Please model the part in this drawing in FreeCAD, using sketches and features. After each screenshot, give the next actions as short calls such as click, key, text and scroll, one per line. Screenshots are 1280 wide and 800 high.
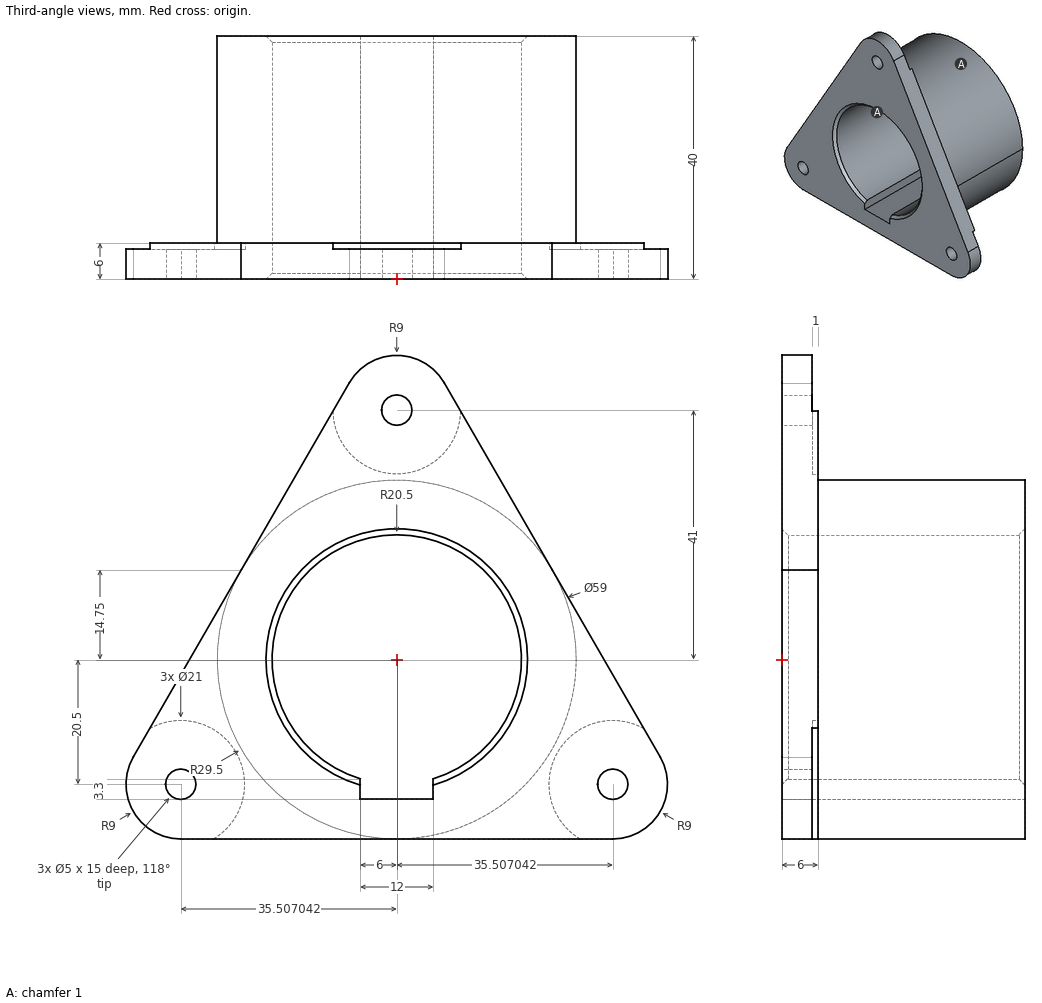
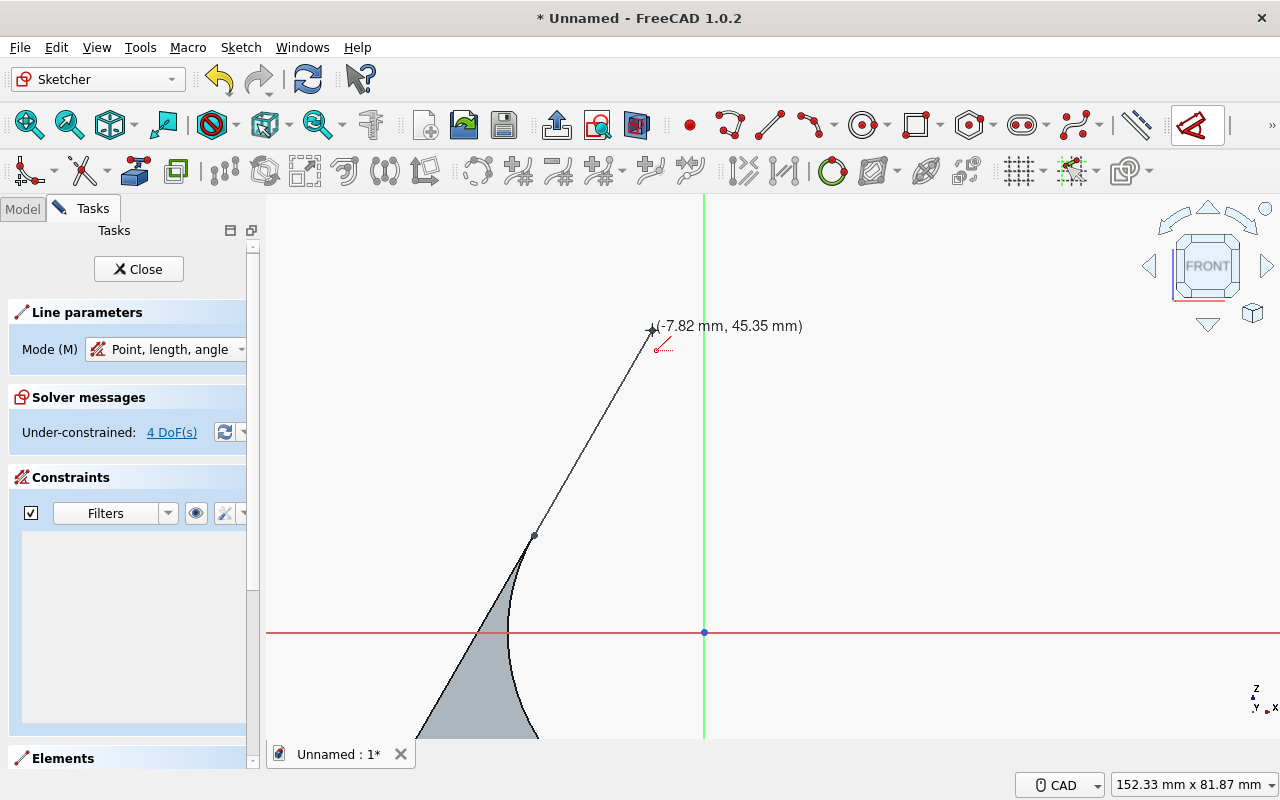
click(756, 330)
click(874, 535)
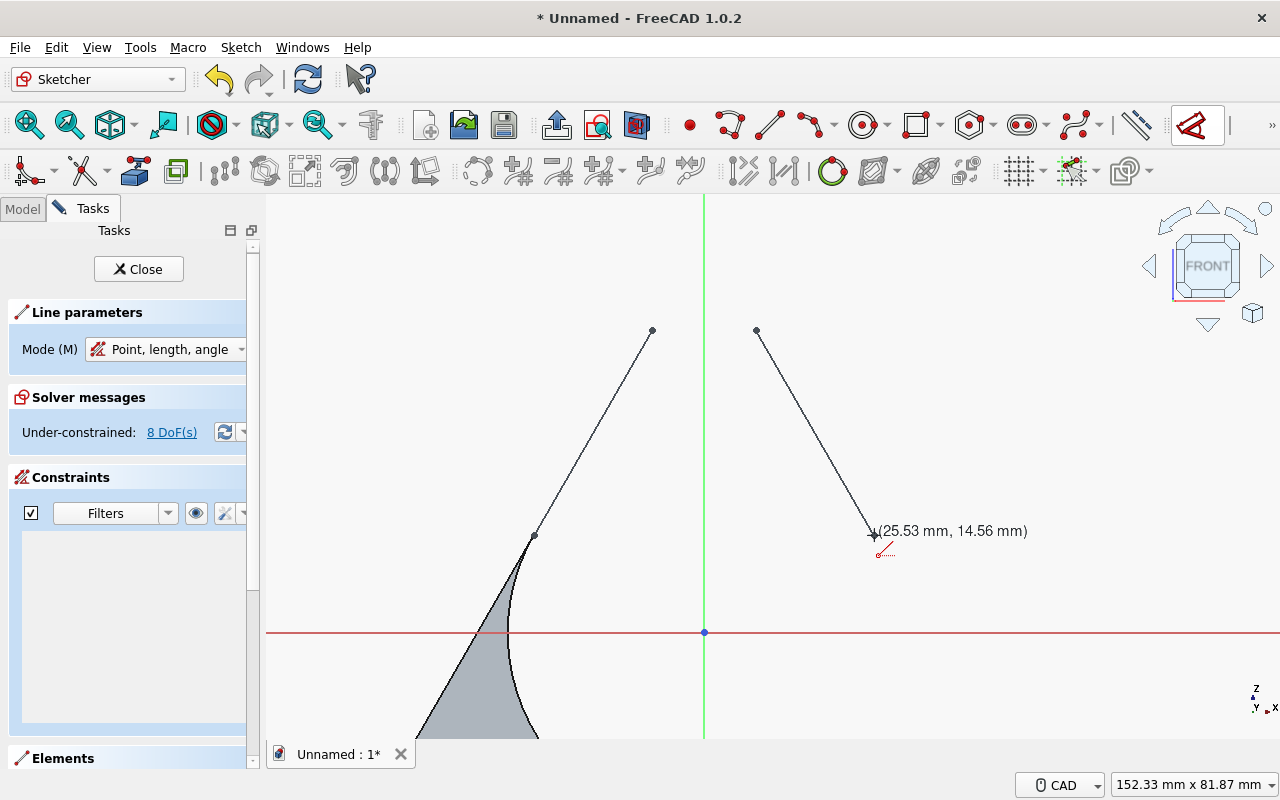
click(810, 126)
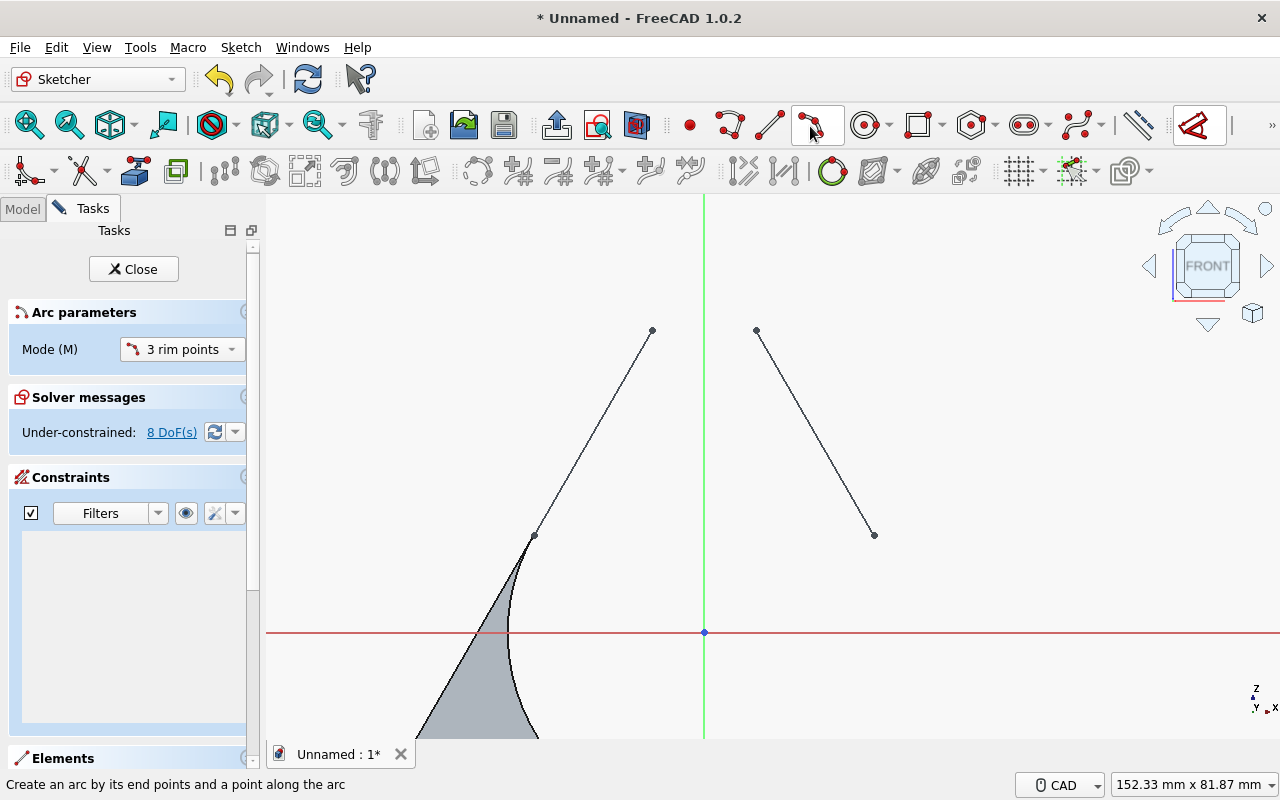
click(652, 331)
click(756, 331)
click(728, 305)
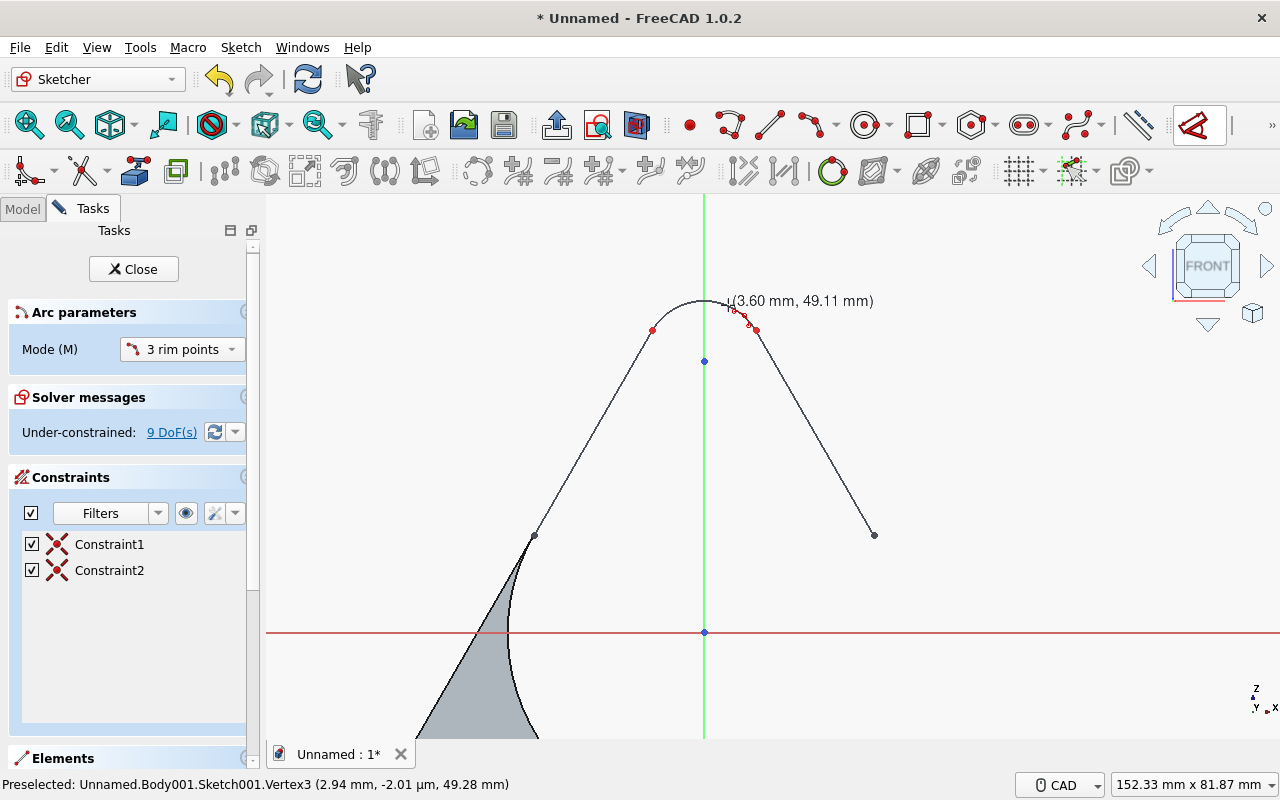
click(874, 536)
click(534, 536)
click(745, 441)
key(Escape)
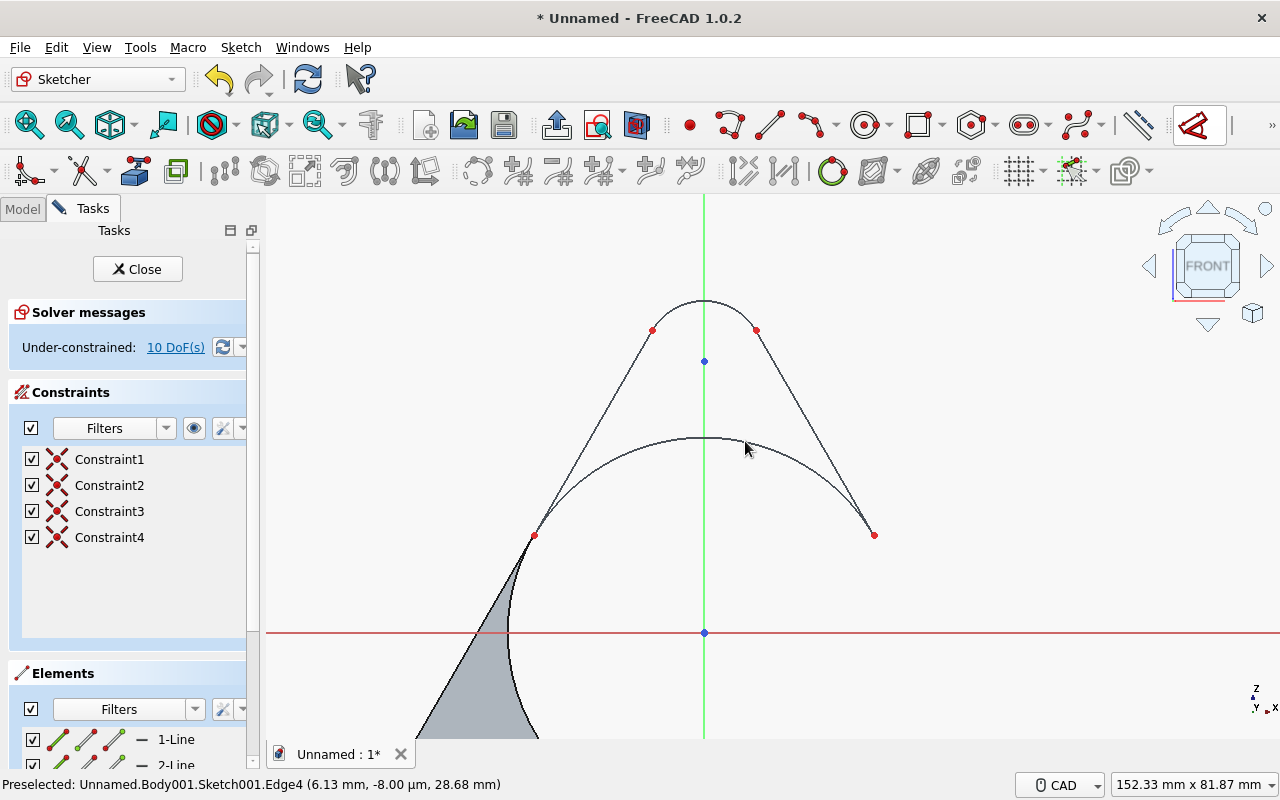
click(569, 474)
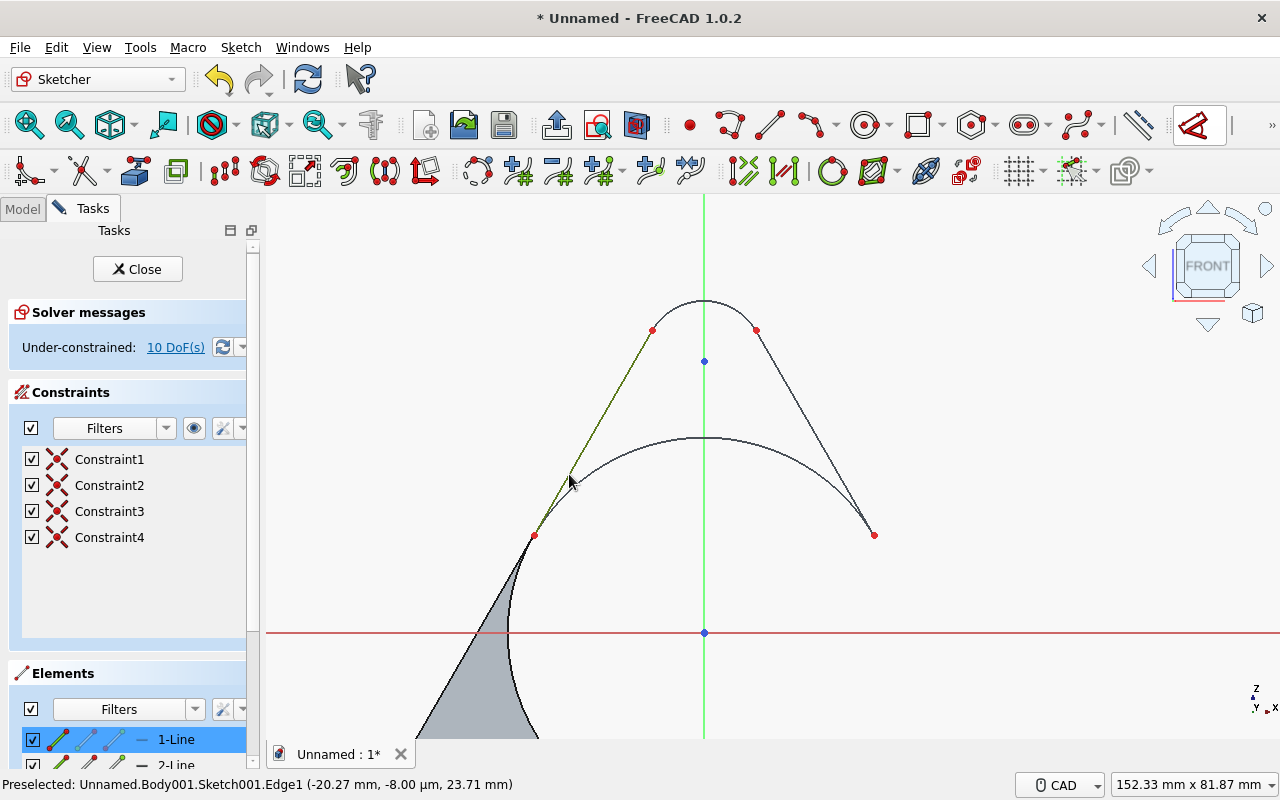
click(728, 306)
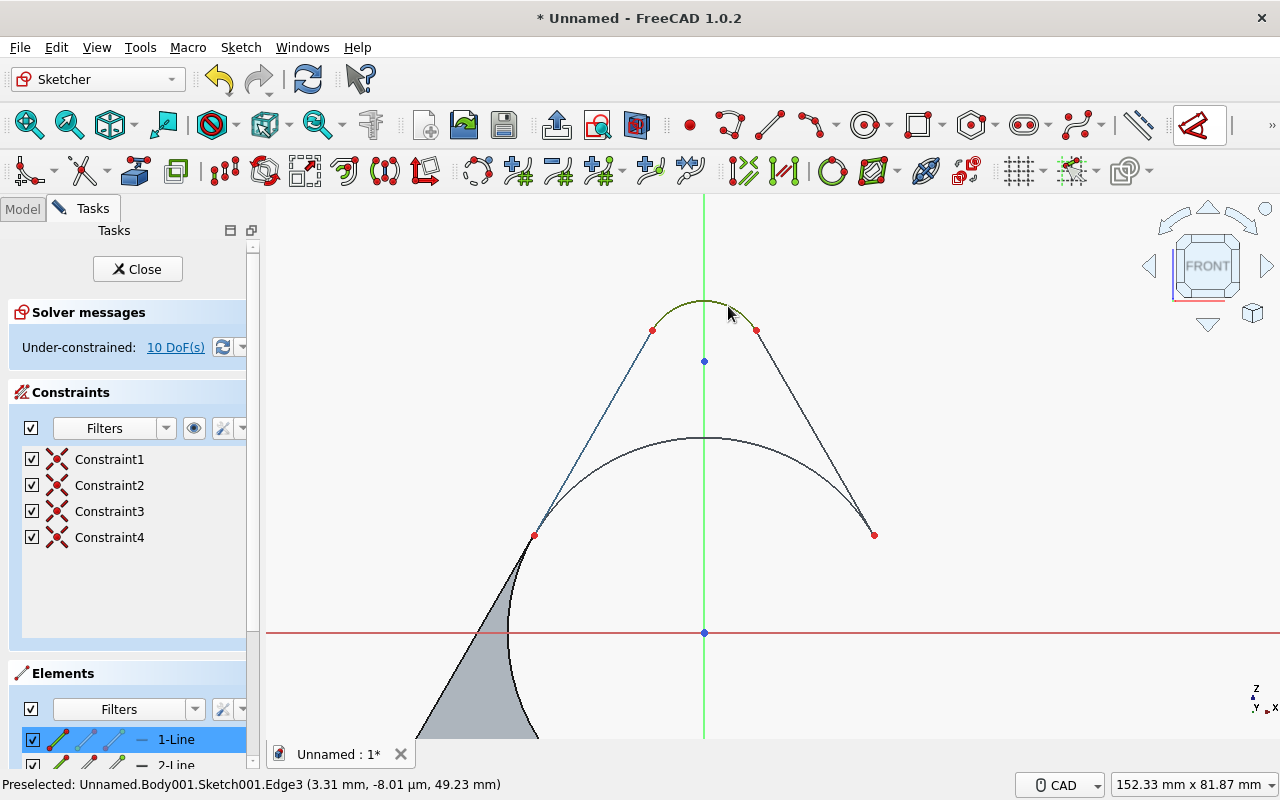
key(t)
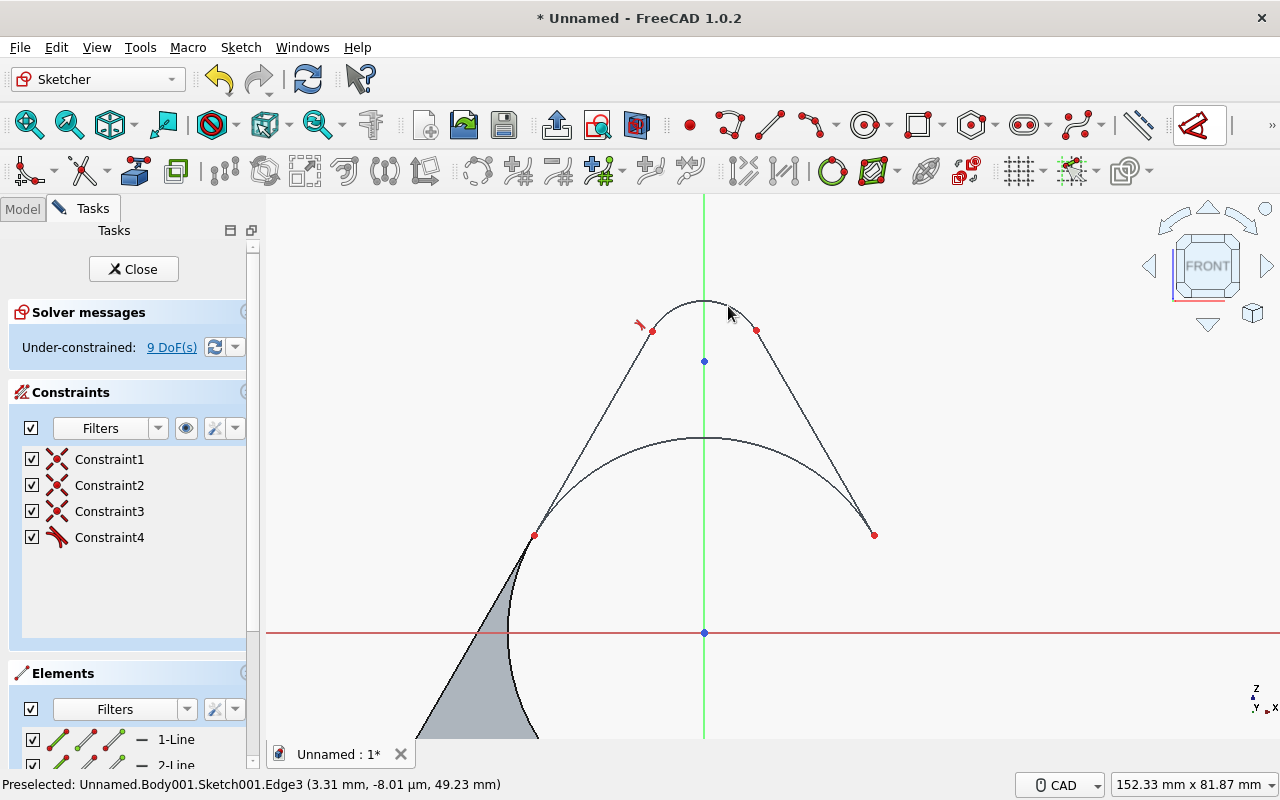
click(569, 475)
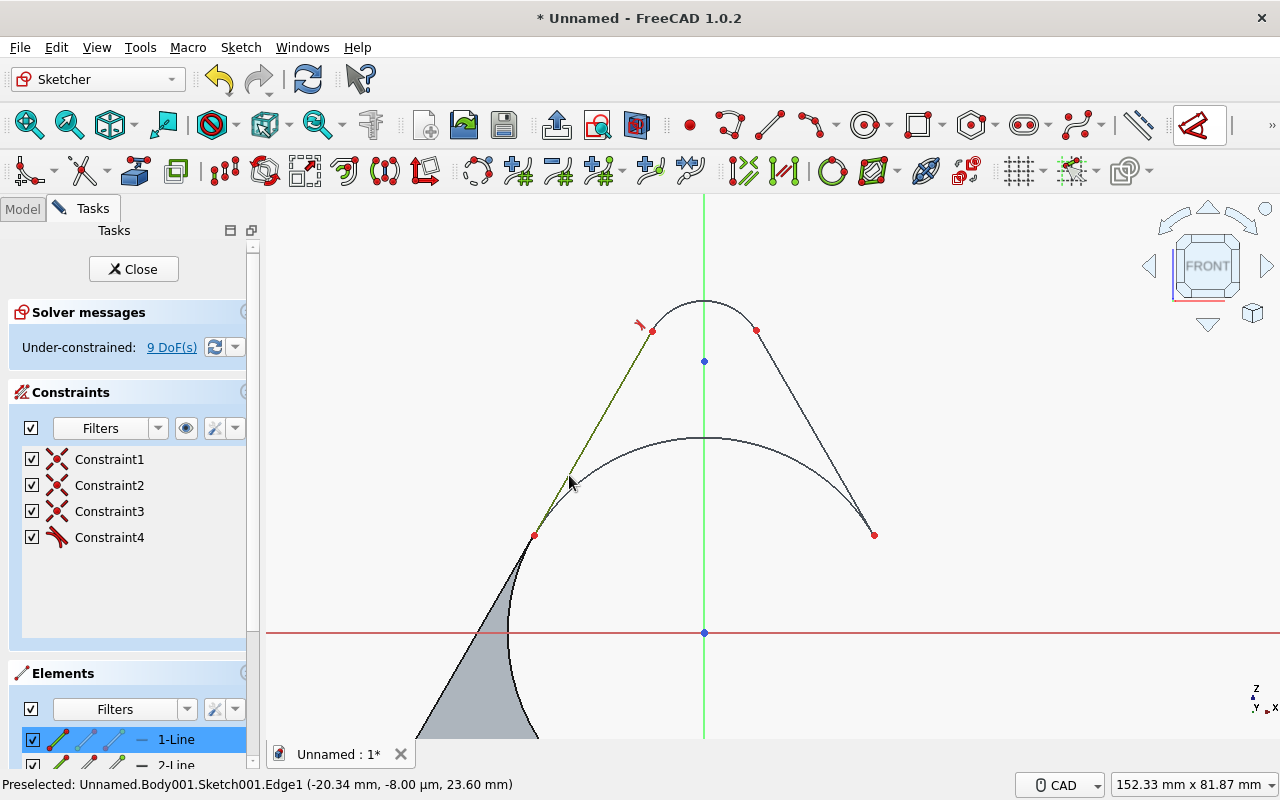
click(784, 455)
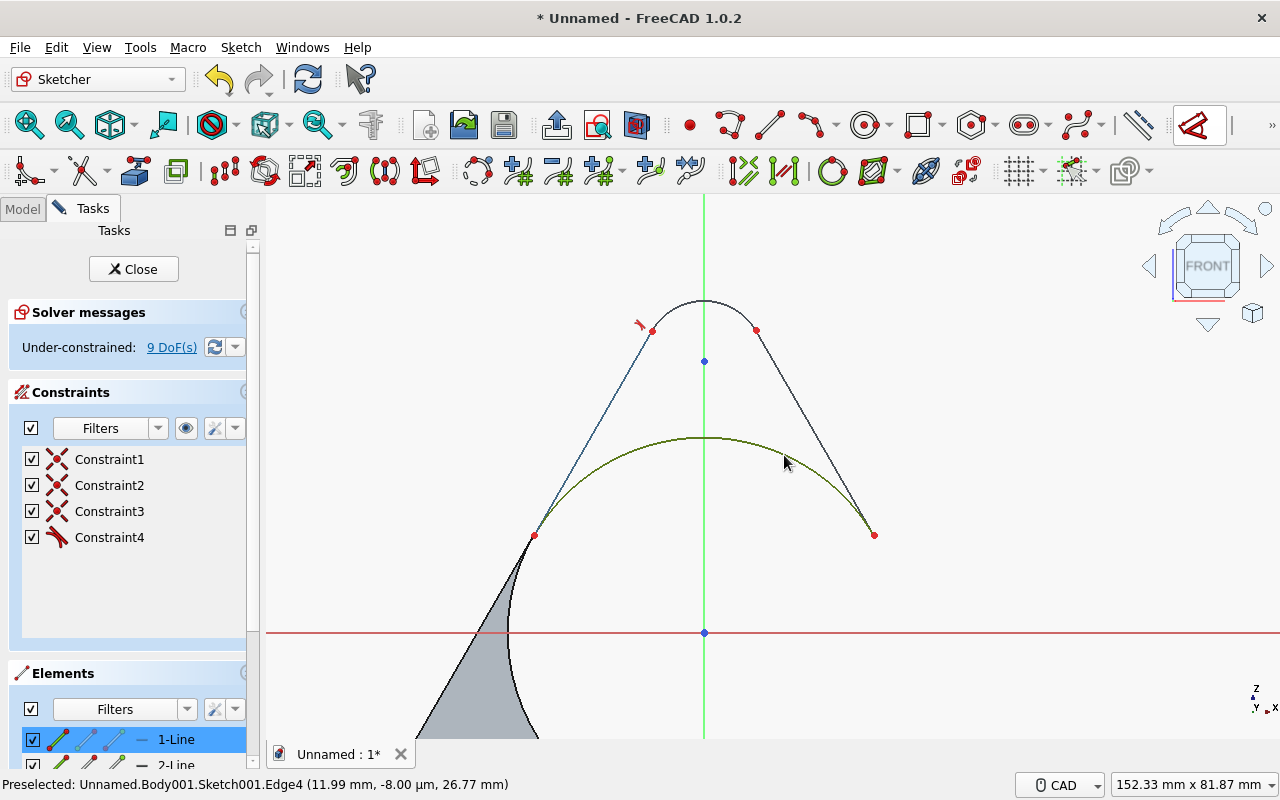
key(t)